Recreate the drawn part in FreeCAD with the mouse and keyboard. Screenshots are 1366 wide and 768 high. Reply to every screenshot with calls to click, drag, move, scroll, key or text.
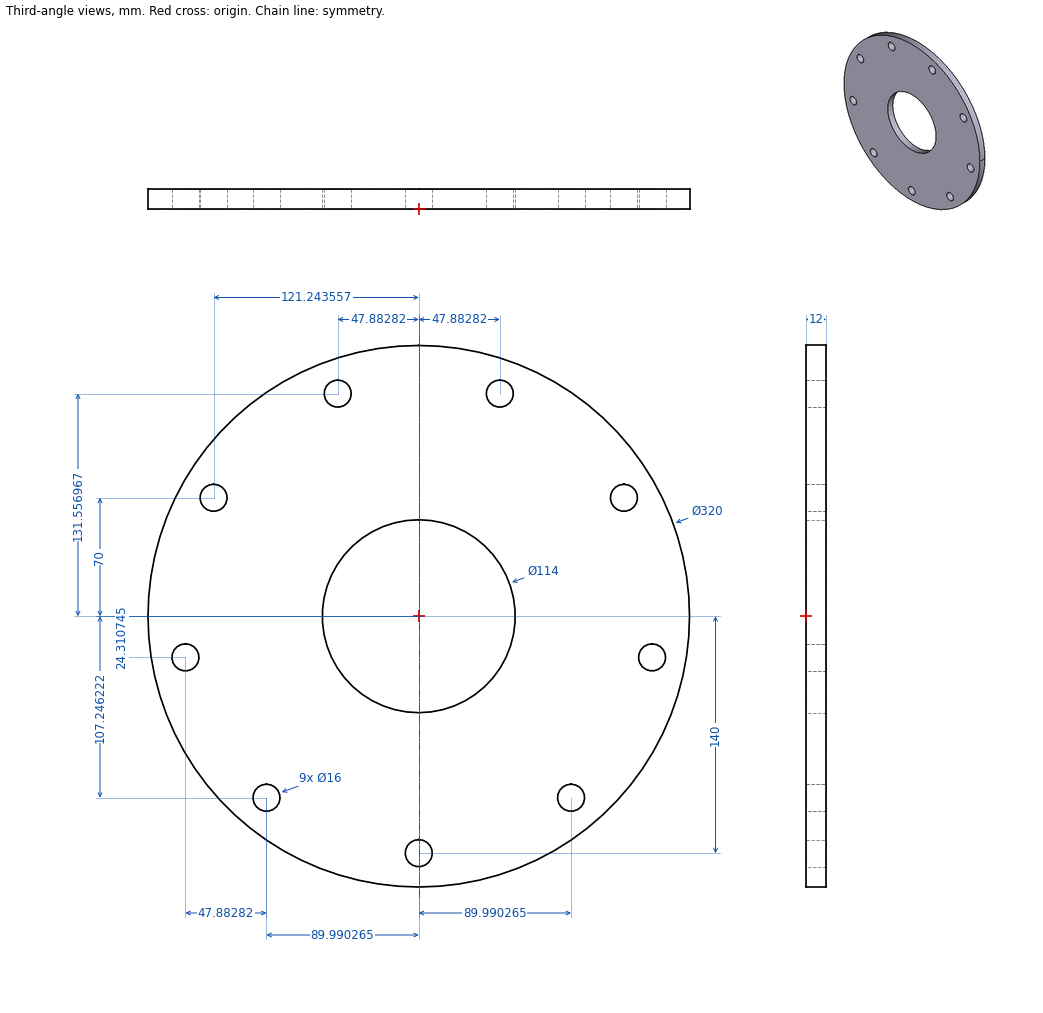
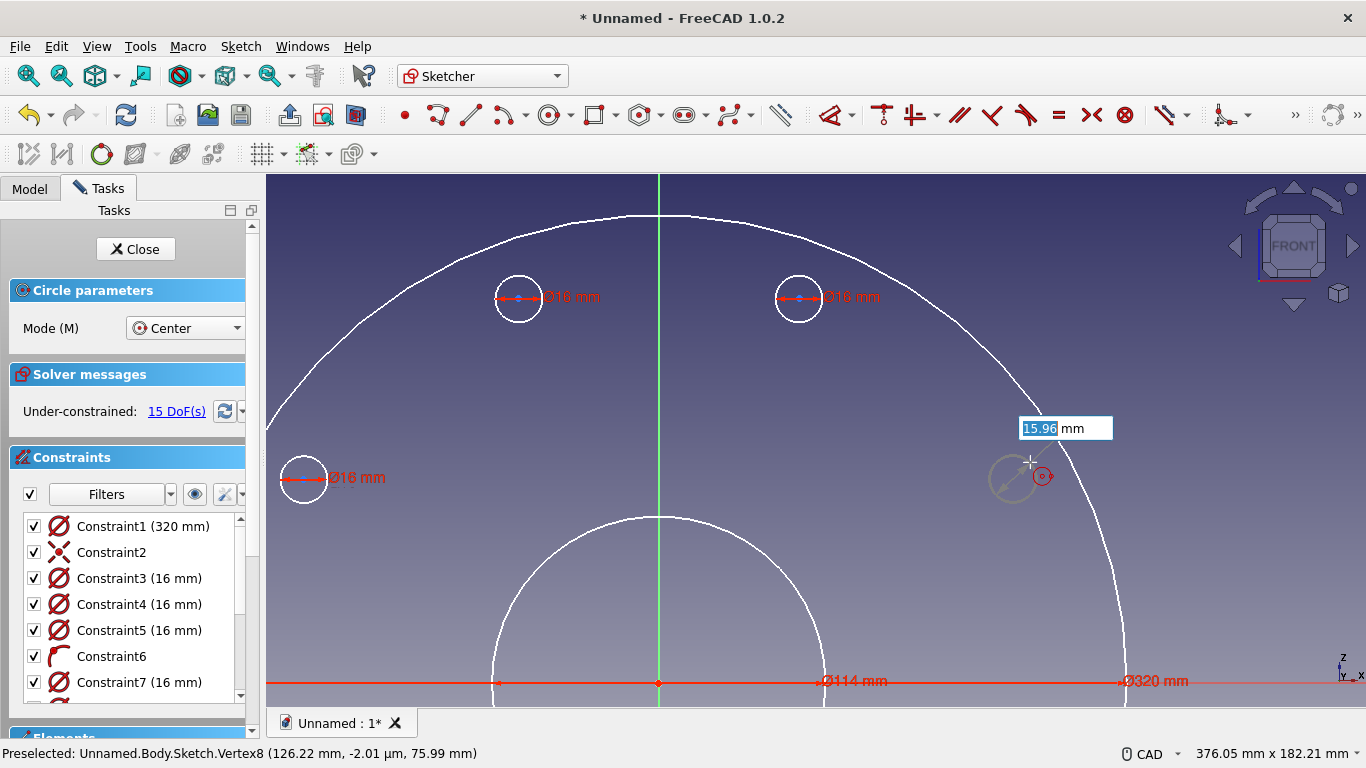
text(16)
key(Return)
key(Escape)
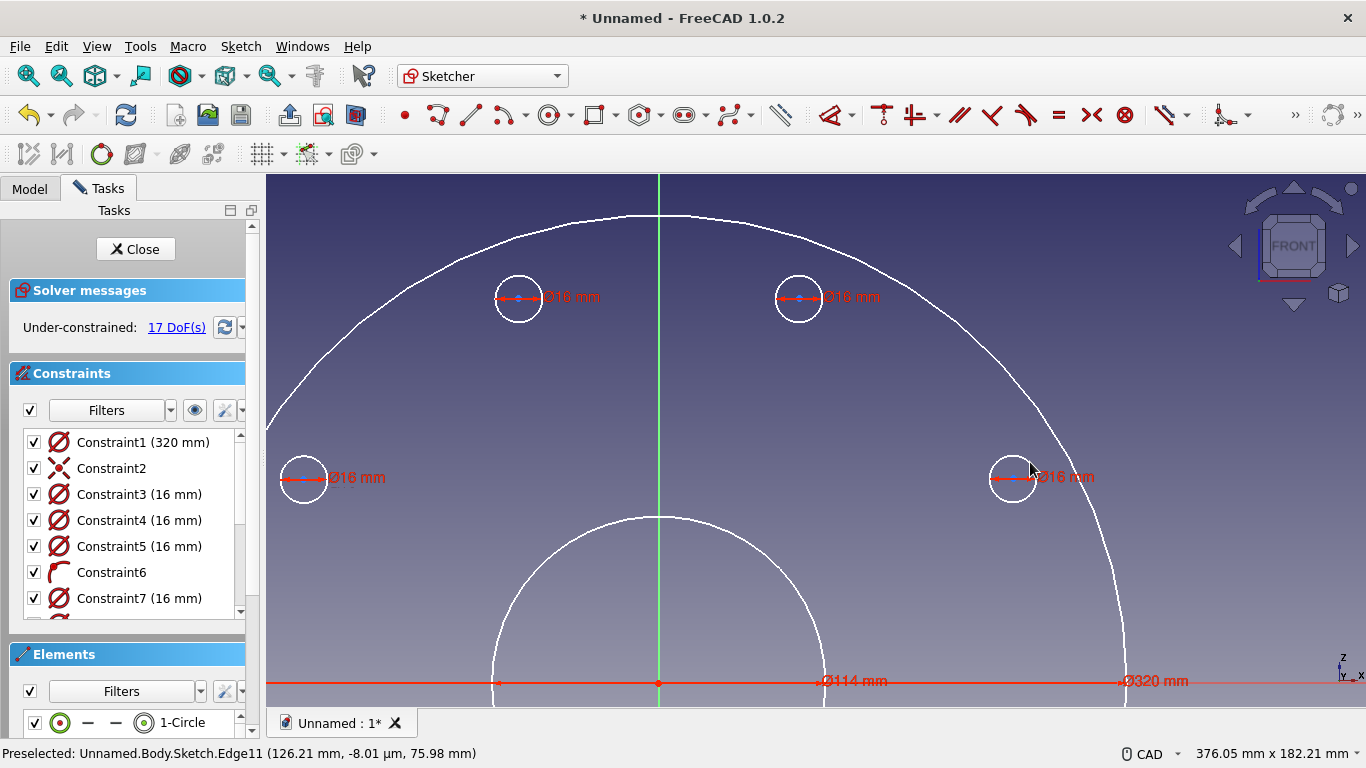
scroll(799, 299, down, 5)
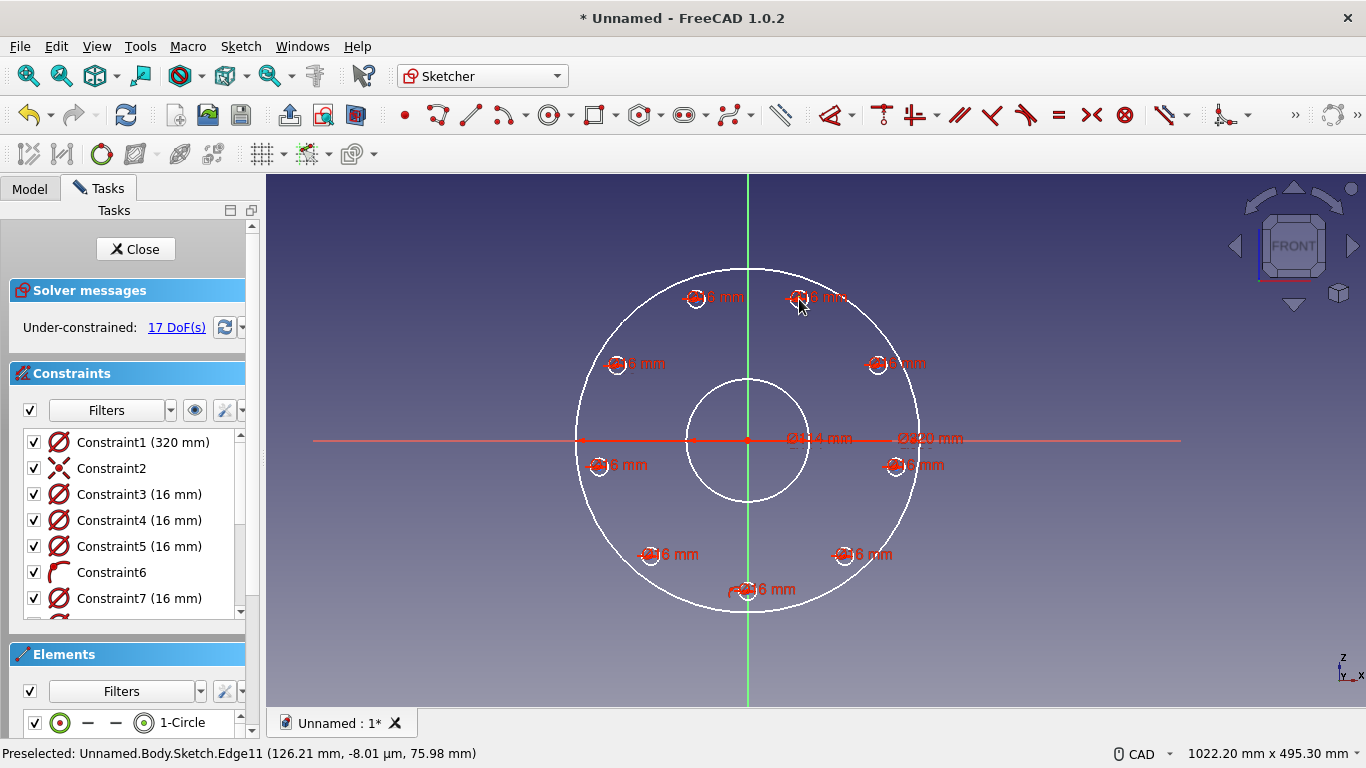
click(651, 556)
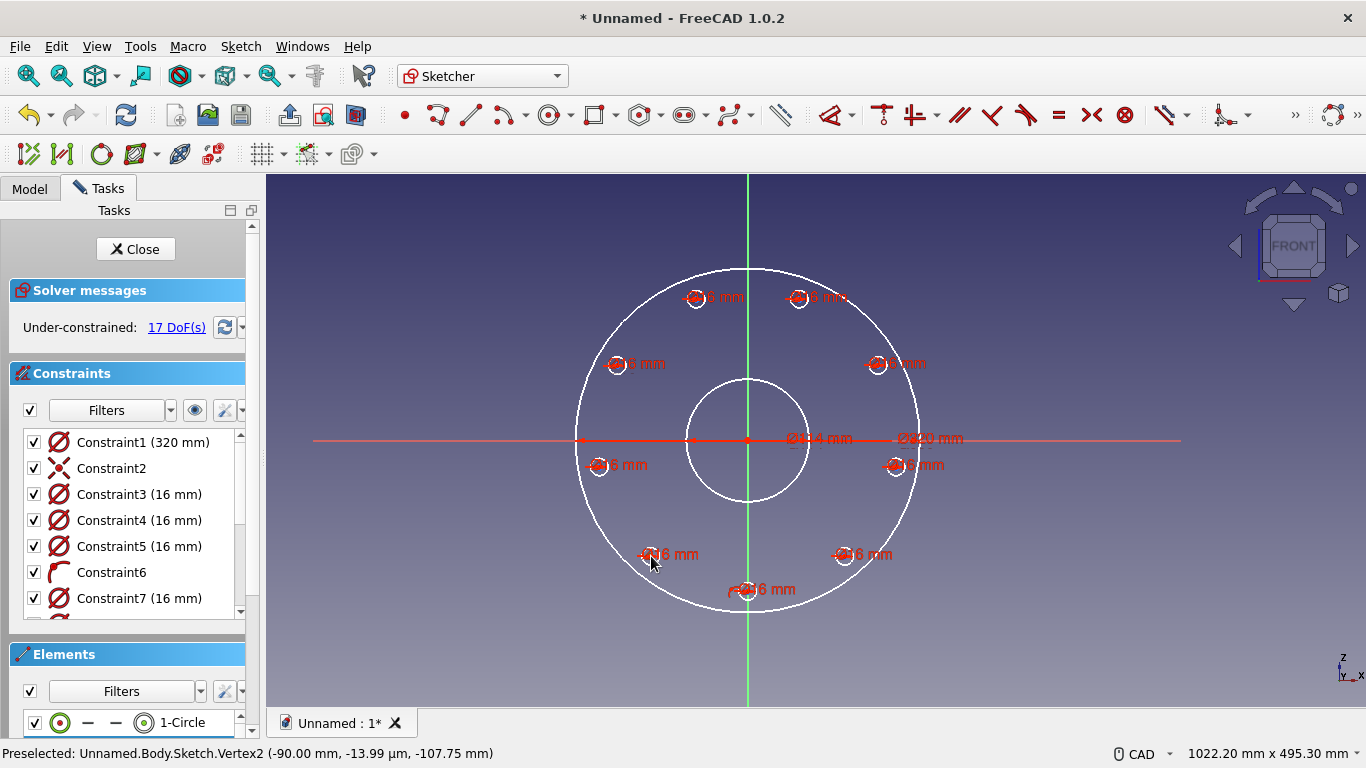
click(845, 556)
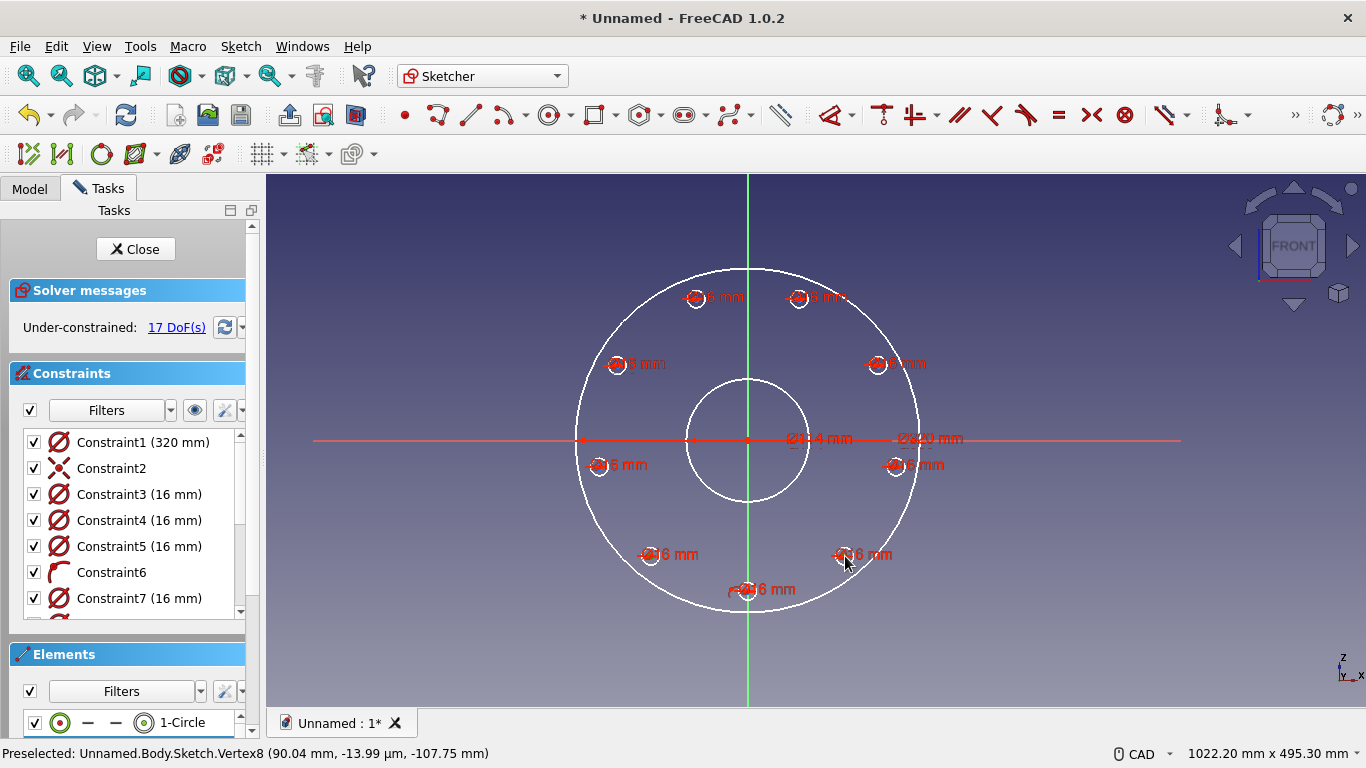
key(h)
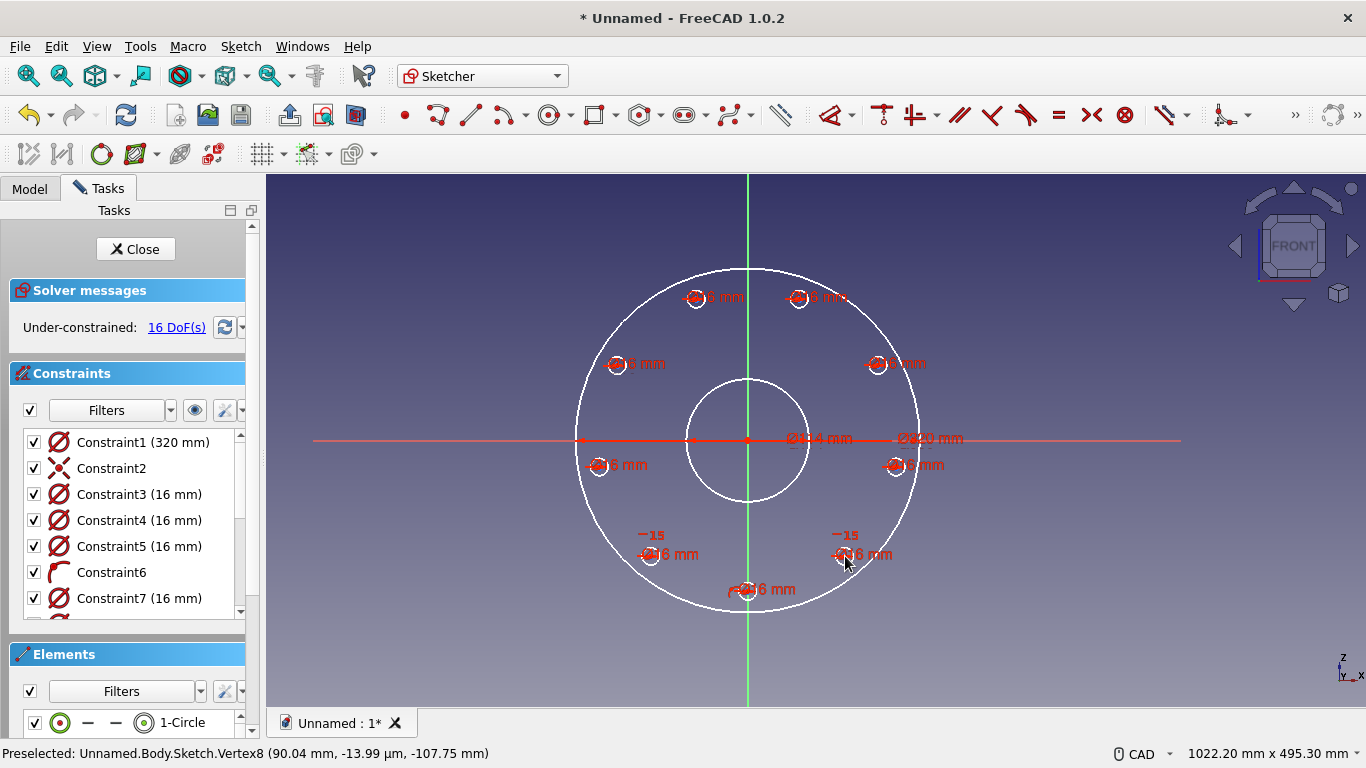
click(696, 299)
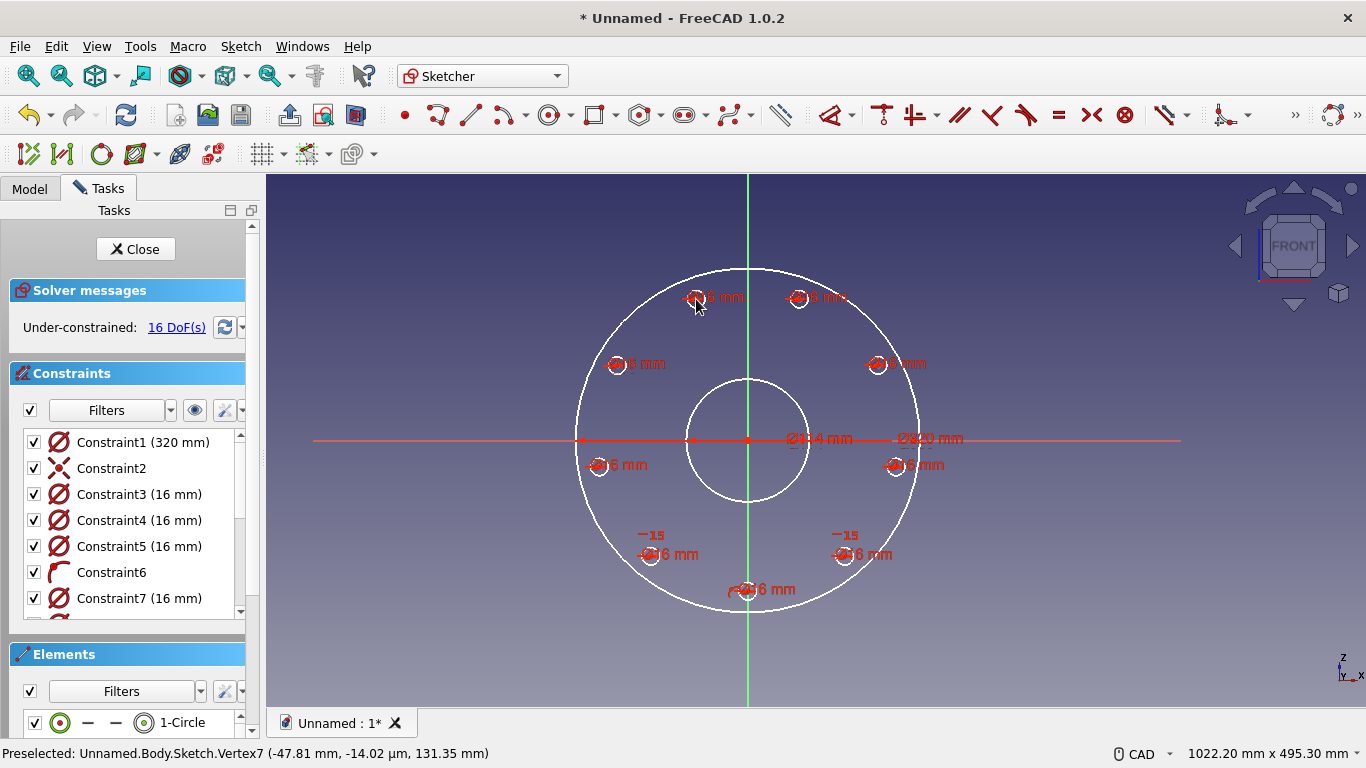
click(799, 299)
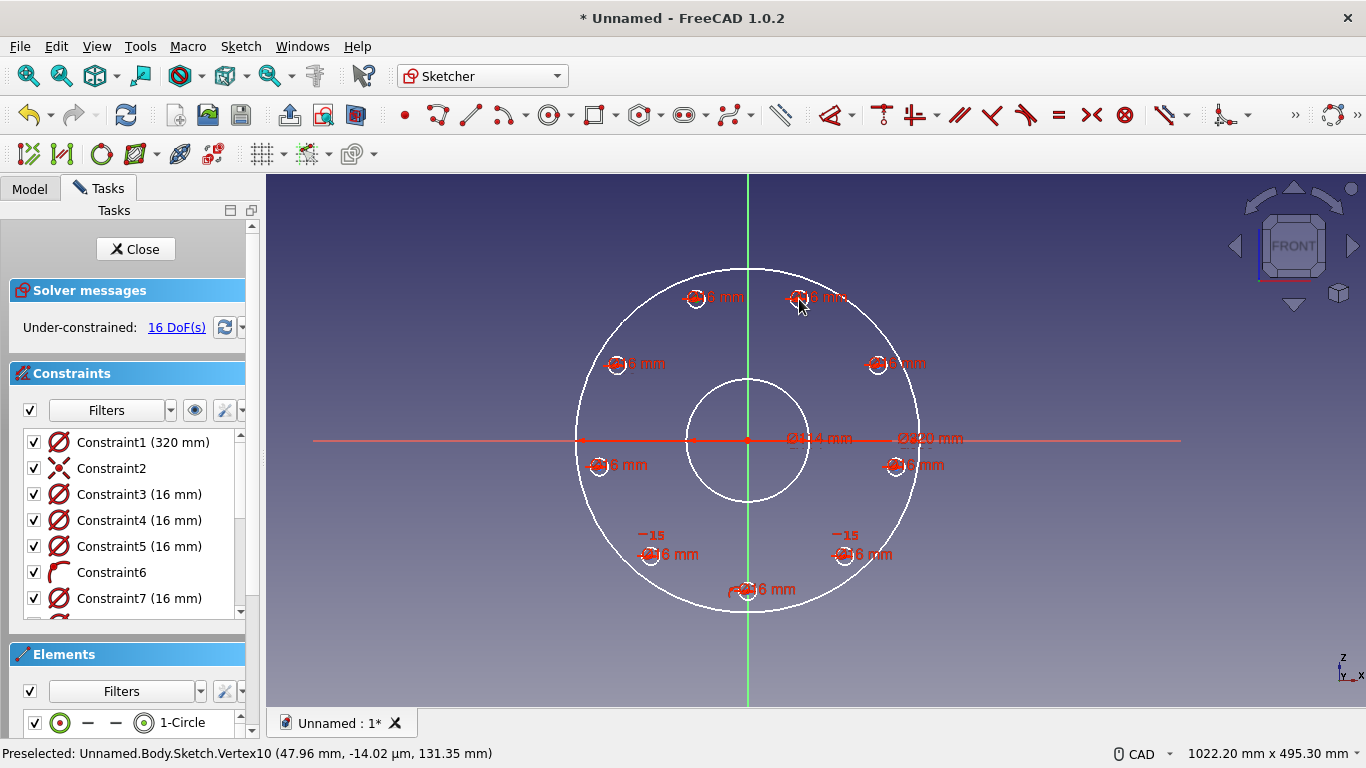
click(936, 116)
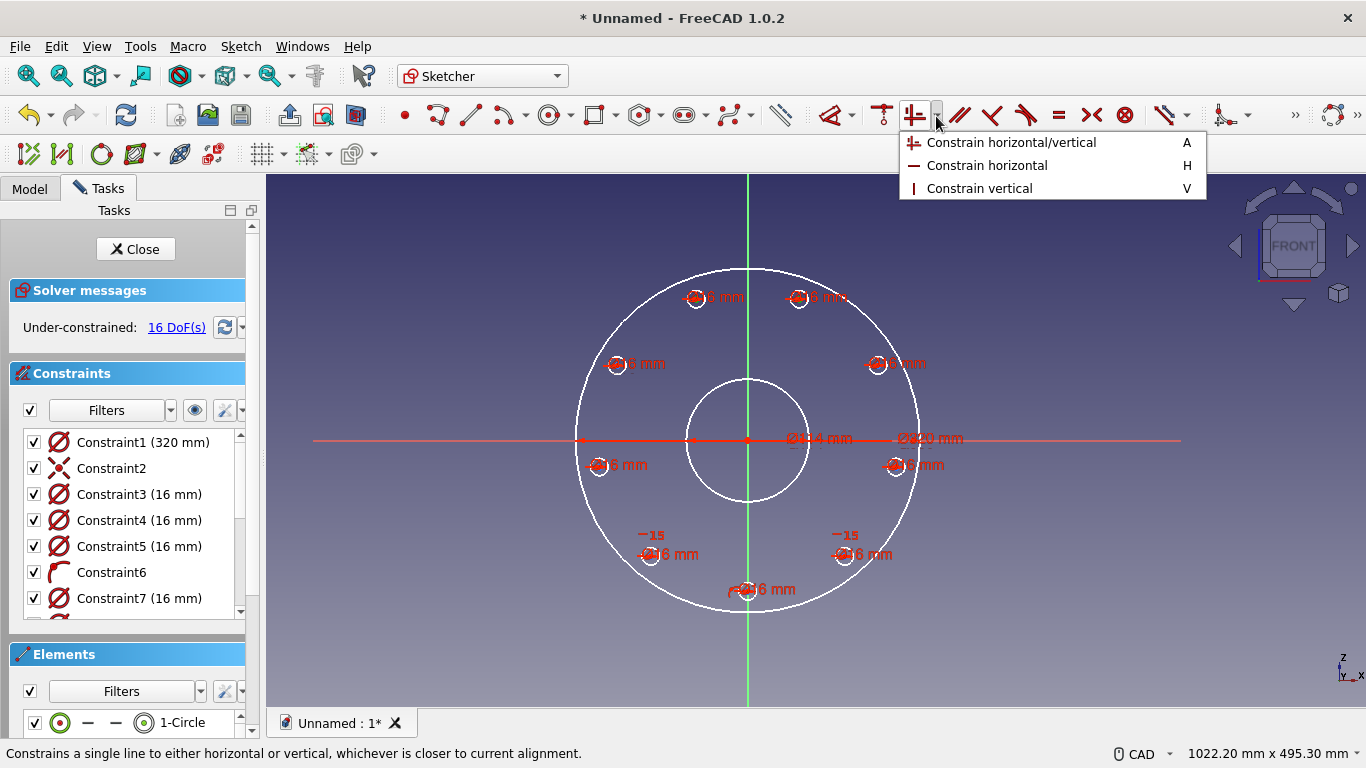
click(1053, 166)